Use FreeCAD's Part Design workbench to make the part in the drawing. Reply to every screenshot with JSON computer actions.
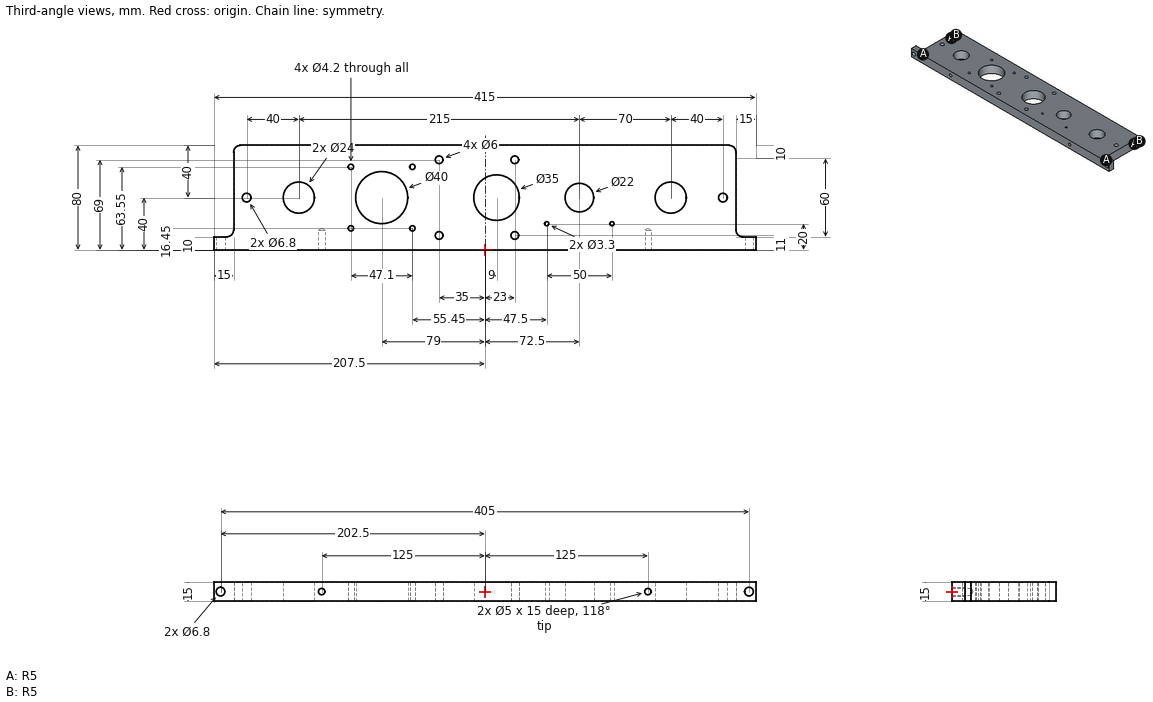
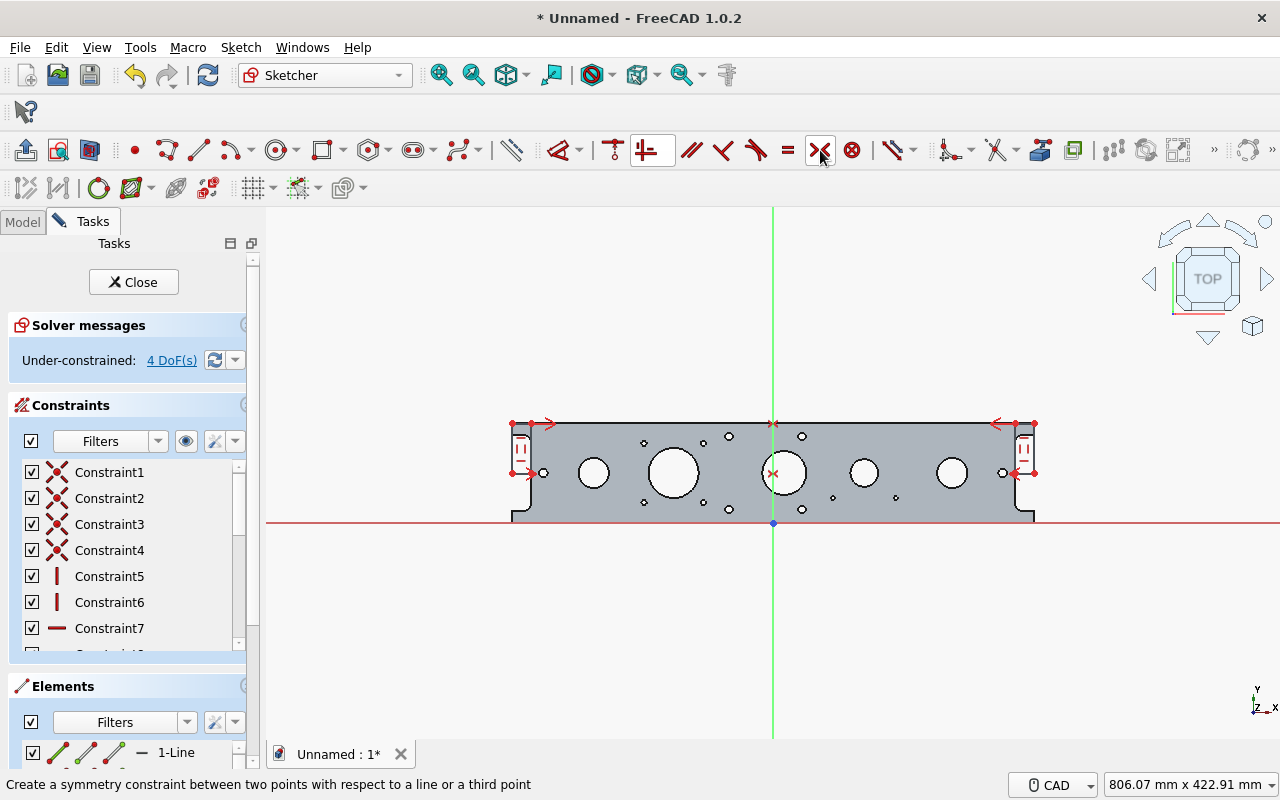
{"action": "left_click", "coordinate": [558, 150]}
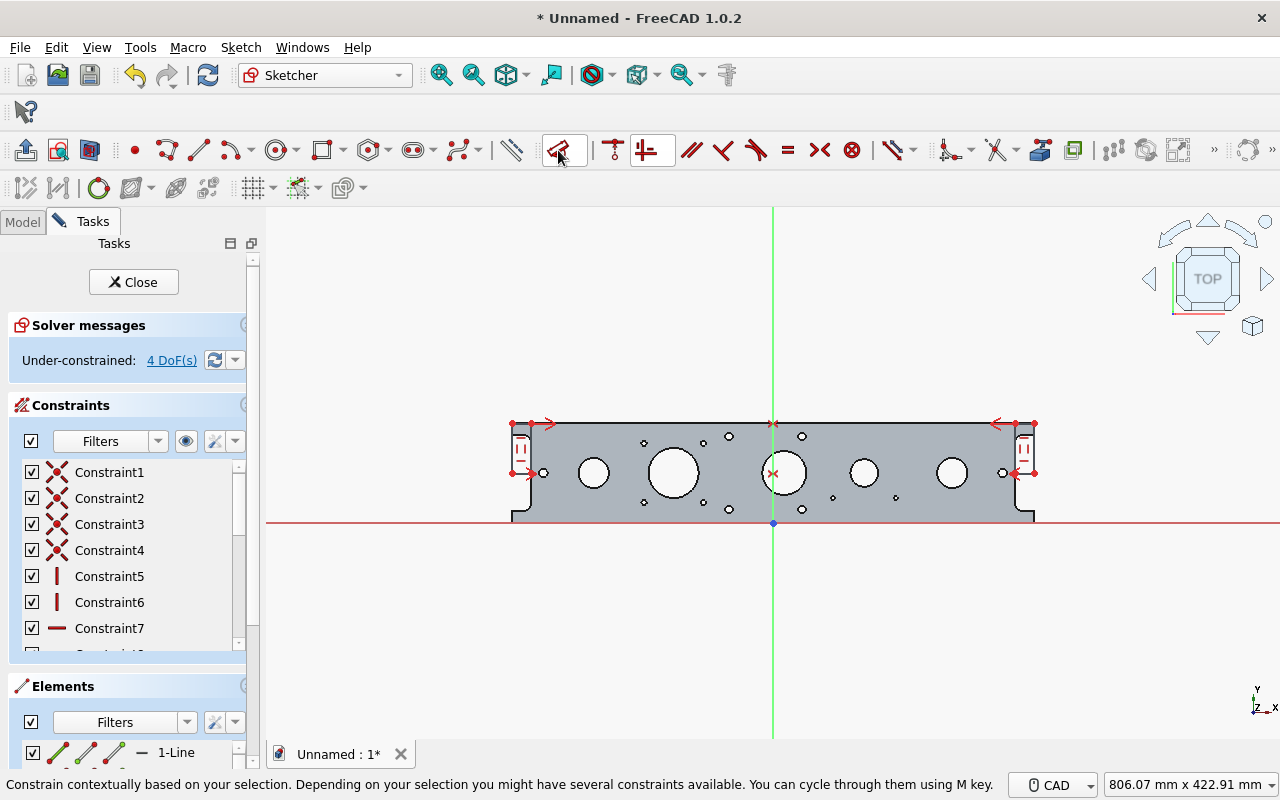
{"action": "left_click", "coordinate": [512, 439]}
{"action": "left_click", "coordinate": [478, 449]}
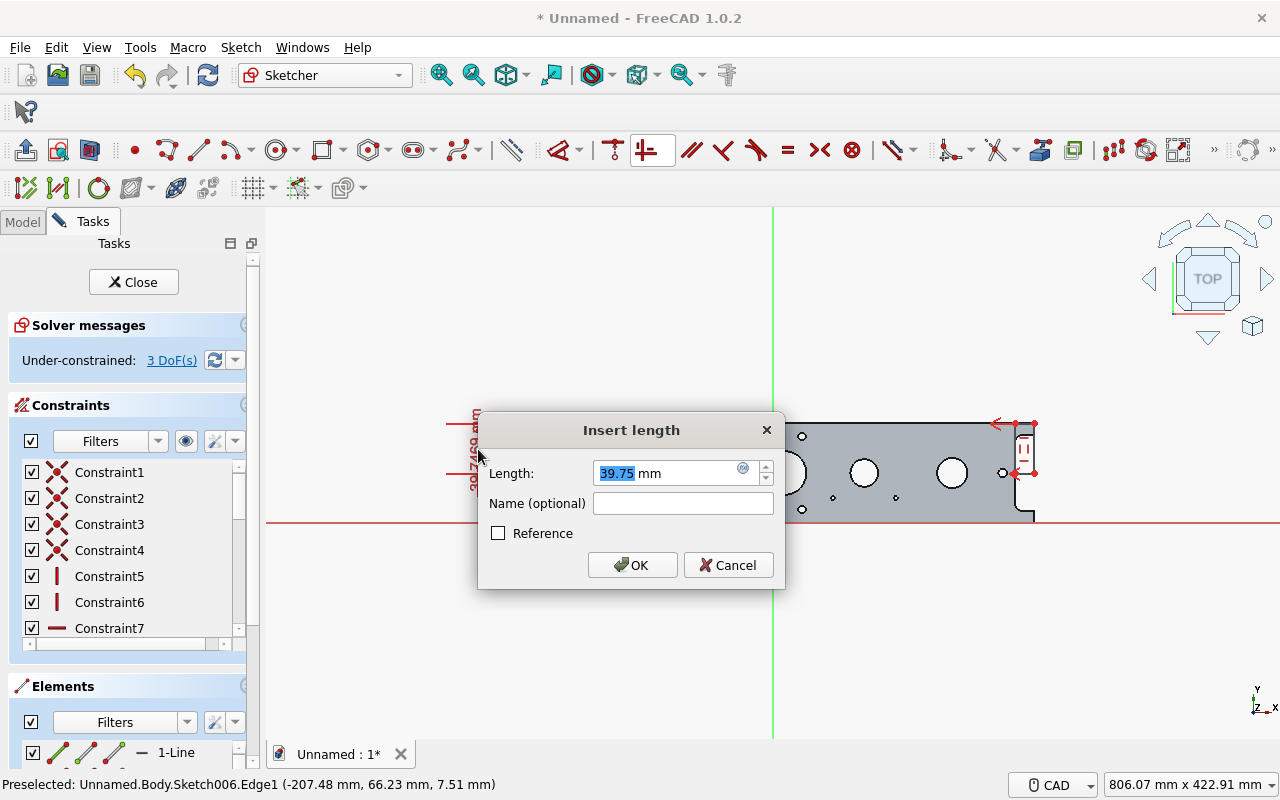
{"action": "type", "text": "40"}
{"action": "key", "text": "Return"}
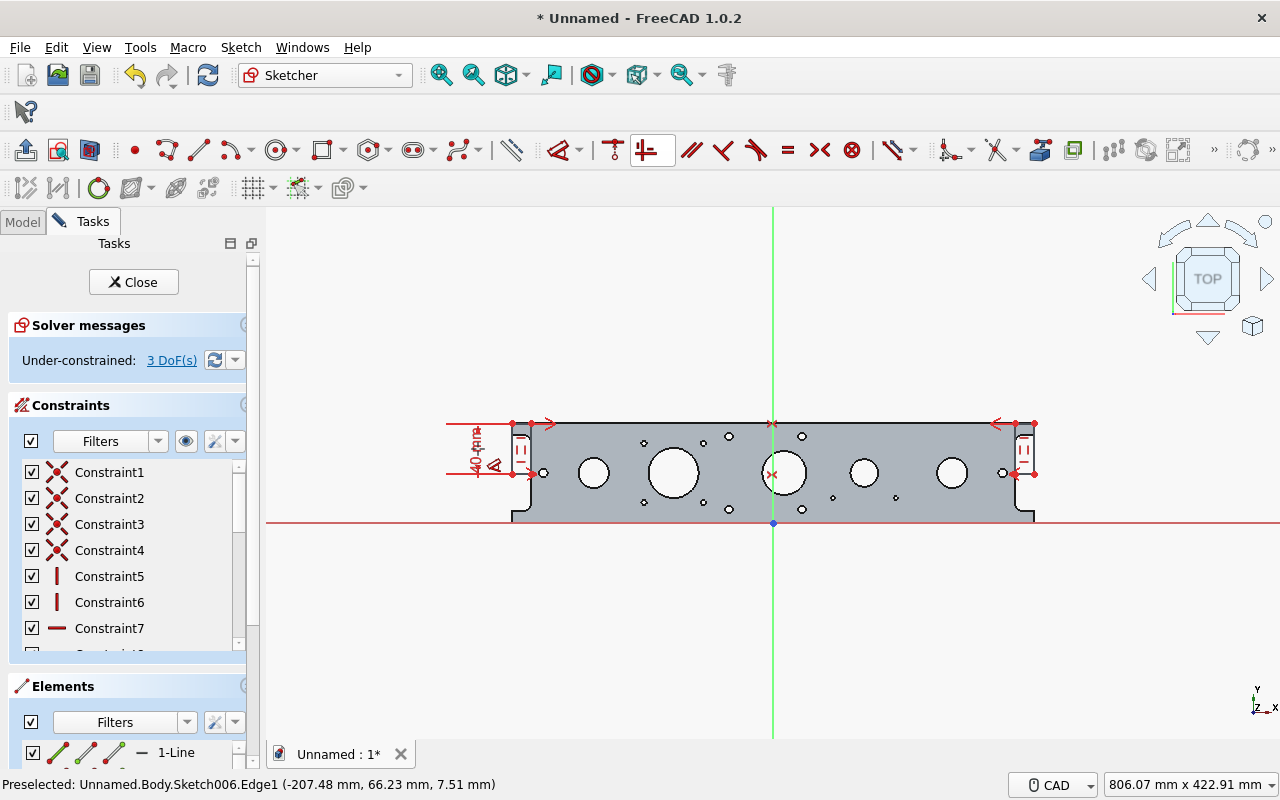
{"action": "scroll", "coordinate": [521, 474], "scroll_direction": "up", "scroll_amount": 4}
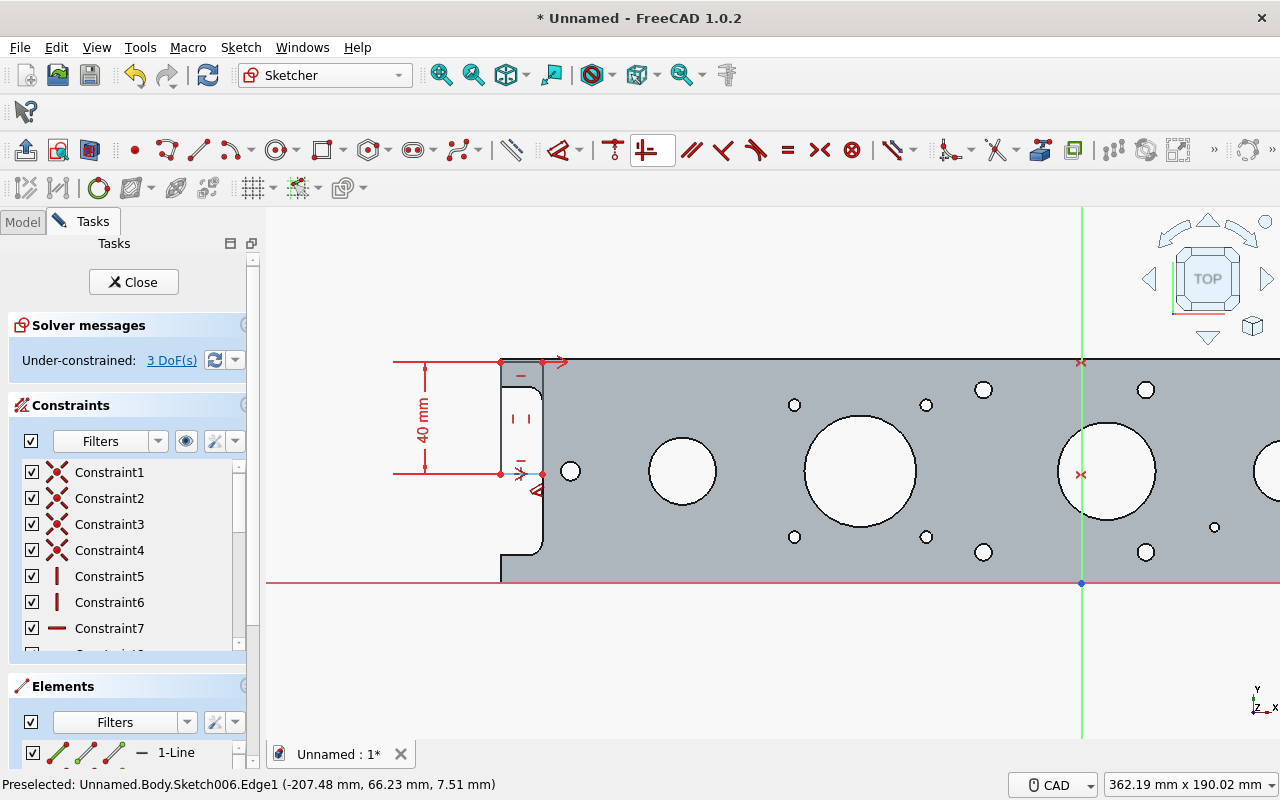
{"action": "left_click", "coordinate": [522, 474]}
{"action": "left_click", "coordinate": [522, 508]}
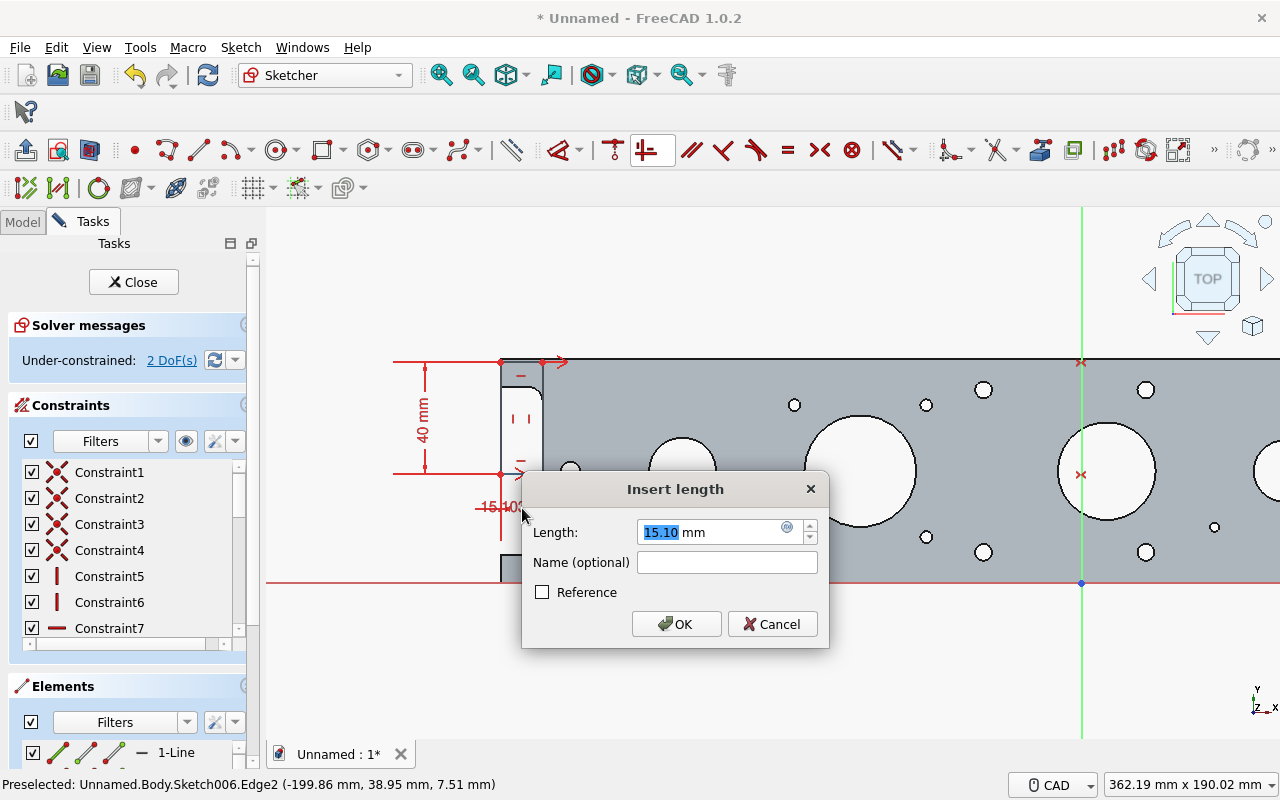
{"action": "type", "text": "15"}
{"action": "key", "text": "Return"}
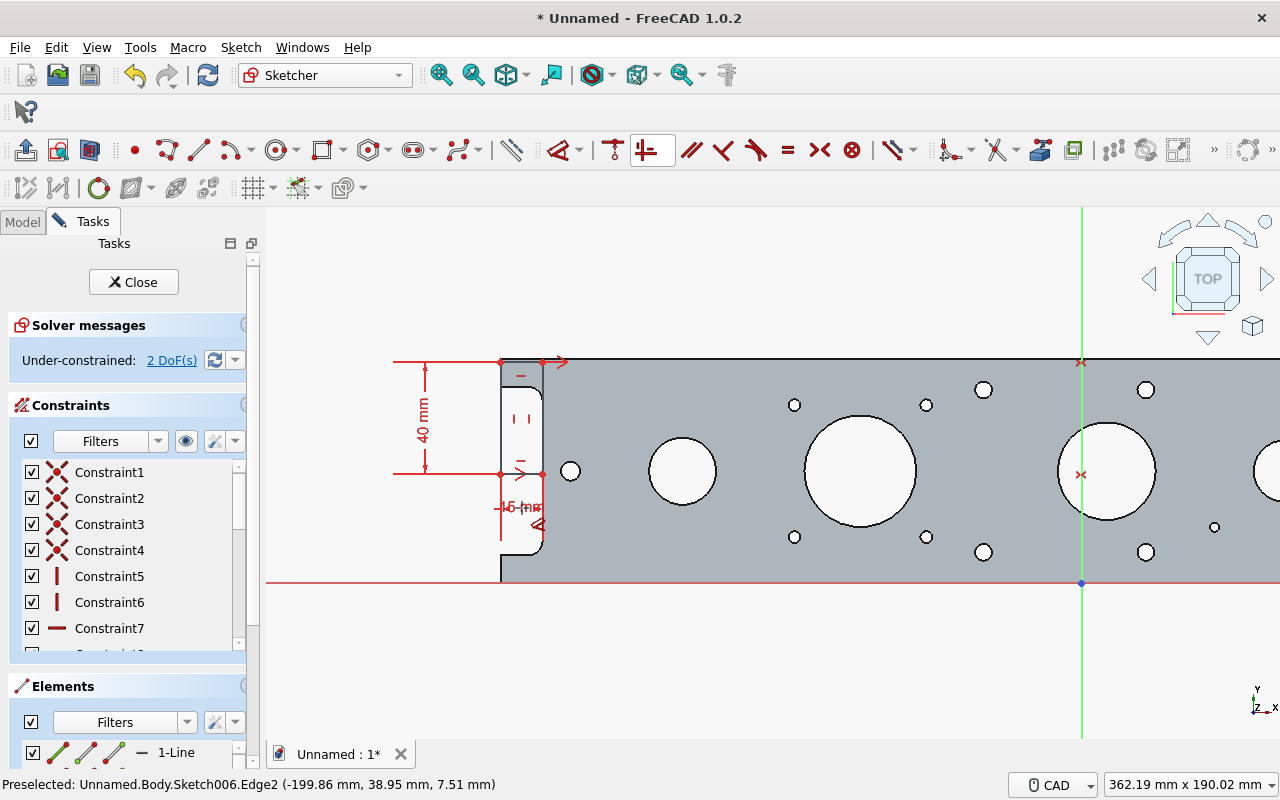
{"action": "left_click", "coordinate": [501, 362]}
{"action": "left_click", "coordinate": [467, 473]}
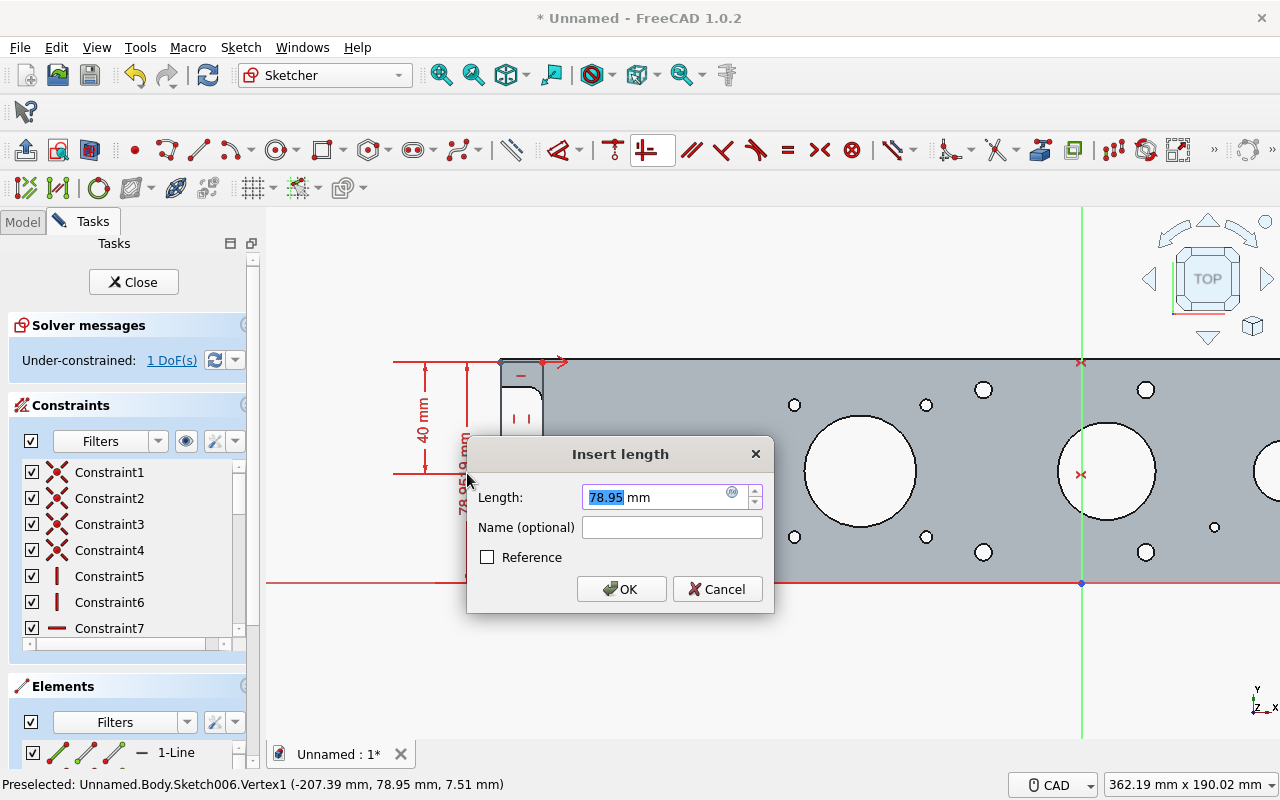
{"action": "type", "text": "80"}
{"action": "key", "text": "Return"}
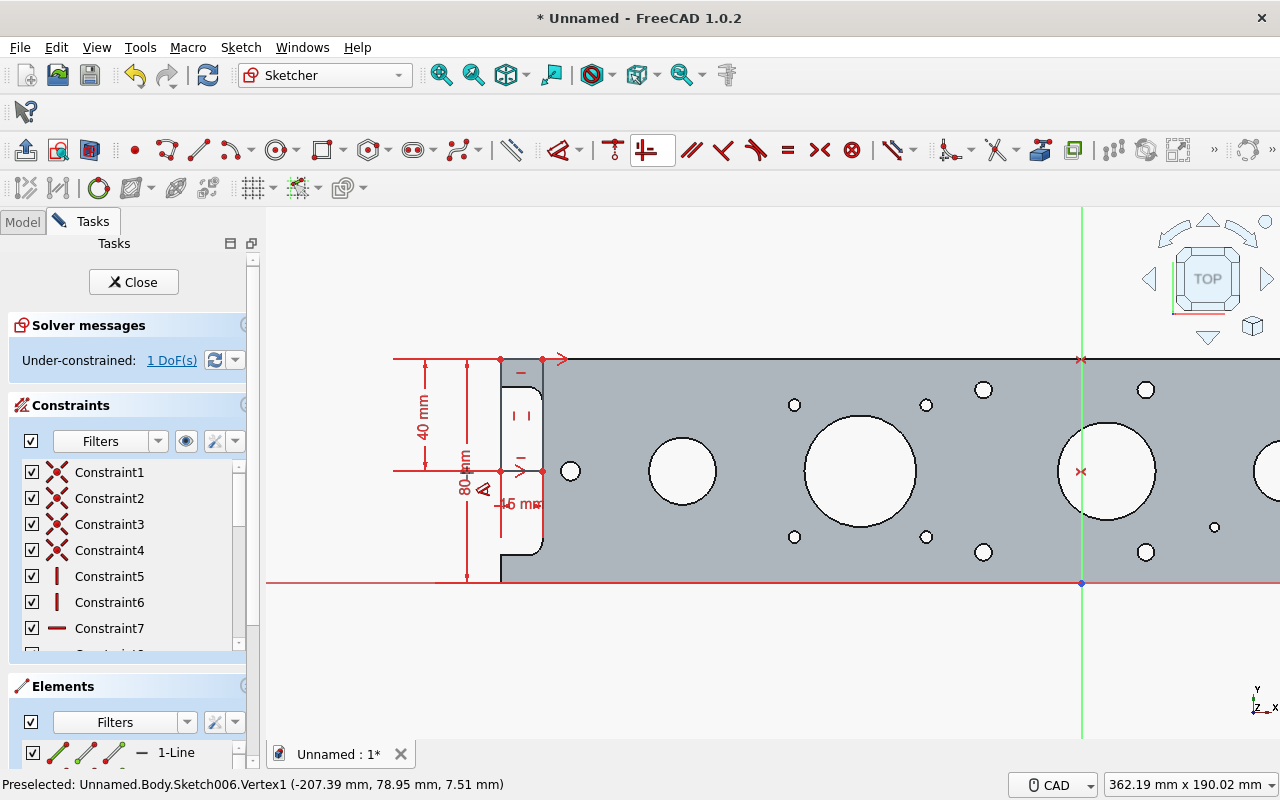
{"action": "left_click", "coordinate": [501, 359]}
{"action": "left_click", "coordinate": [791, 617]}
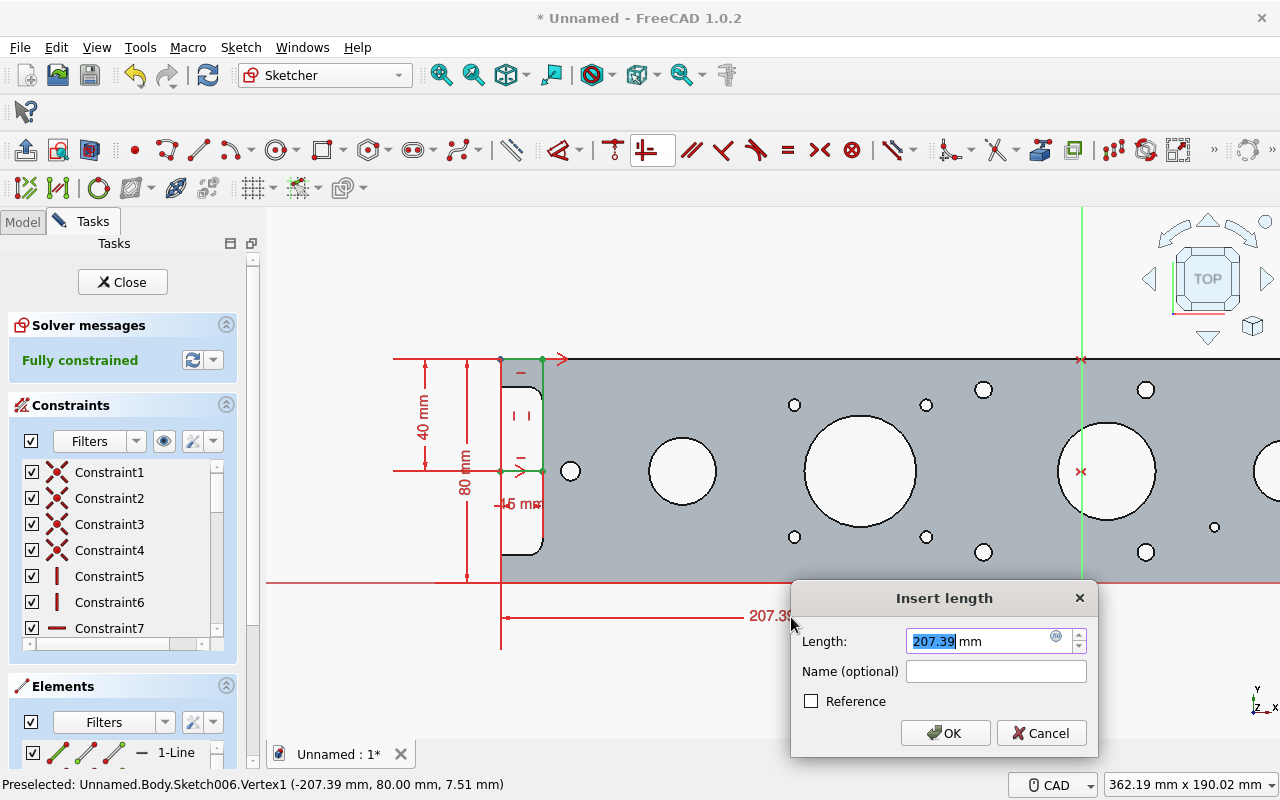
{"action": "type", "text": "207.5"}
{"action": "key", "text": "Return"}
{"action": "key", "text": "Escape"}